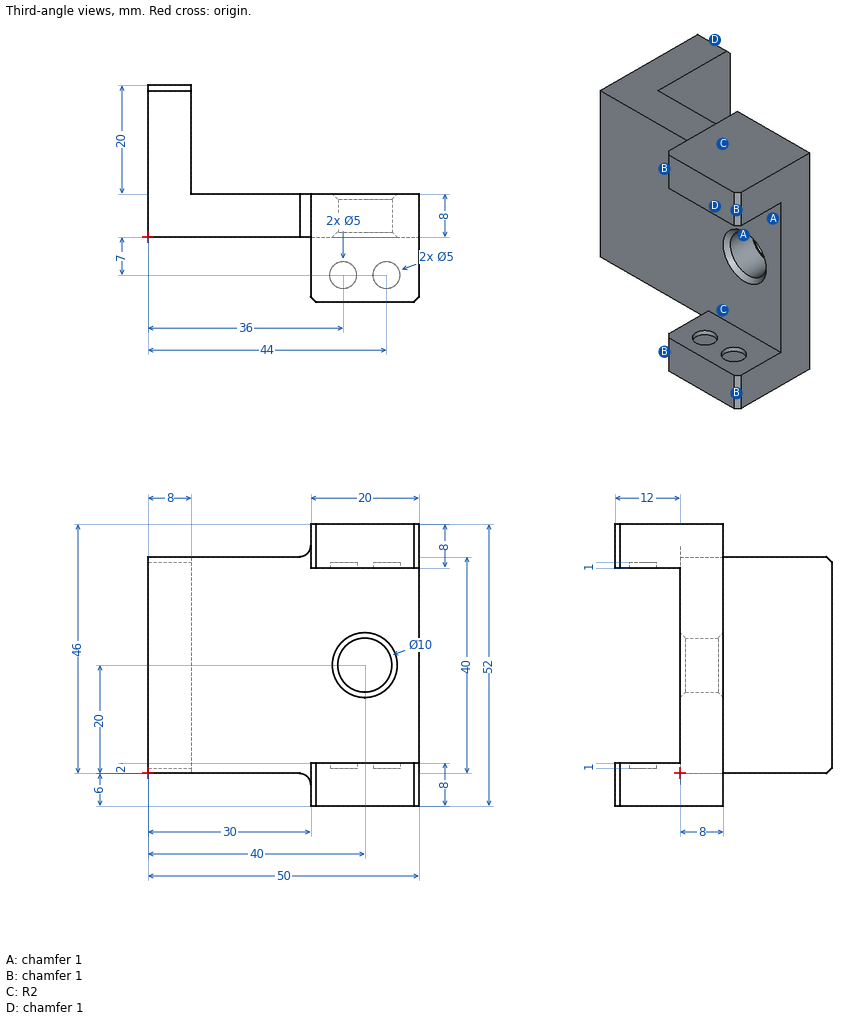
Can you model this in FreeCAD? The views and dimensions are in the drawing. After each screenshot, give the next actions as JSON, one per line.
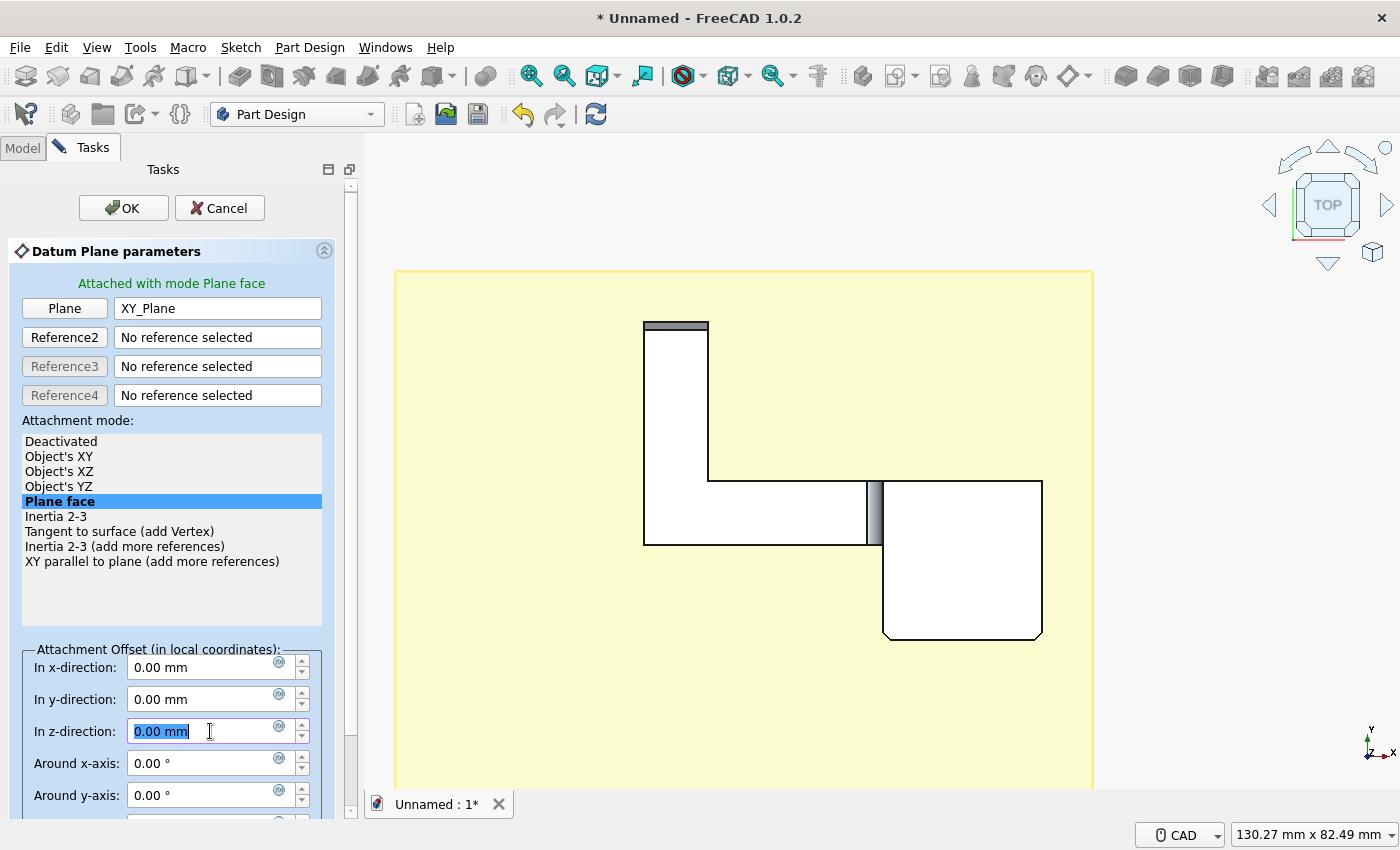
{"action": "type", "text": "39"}
{"action": "key", "text": "Tab"}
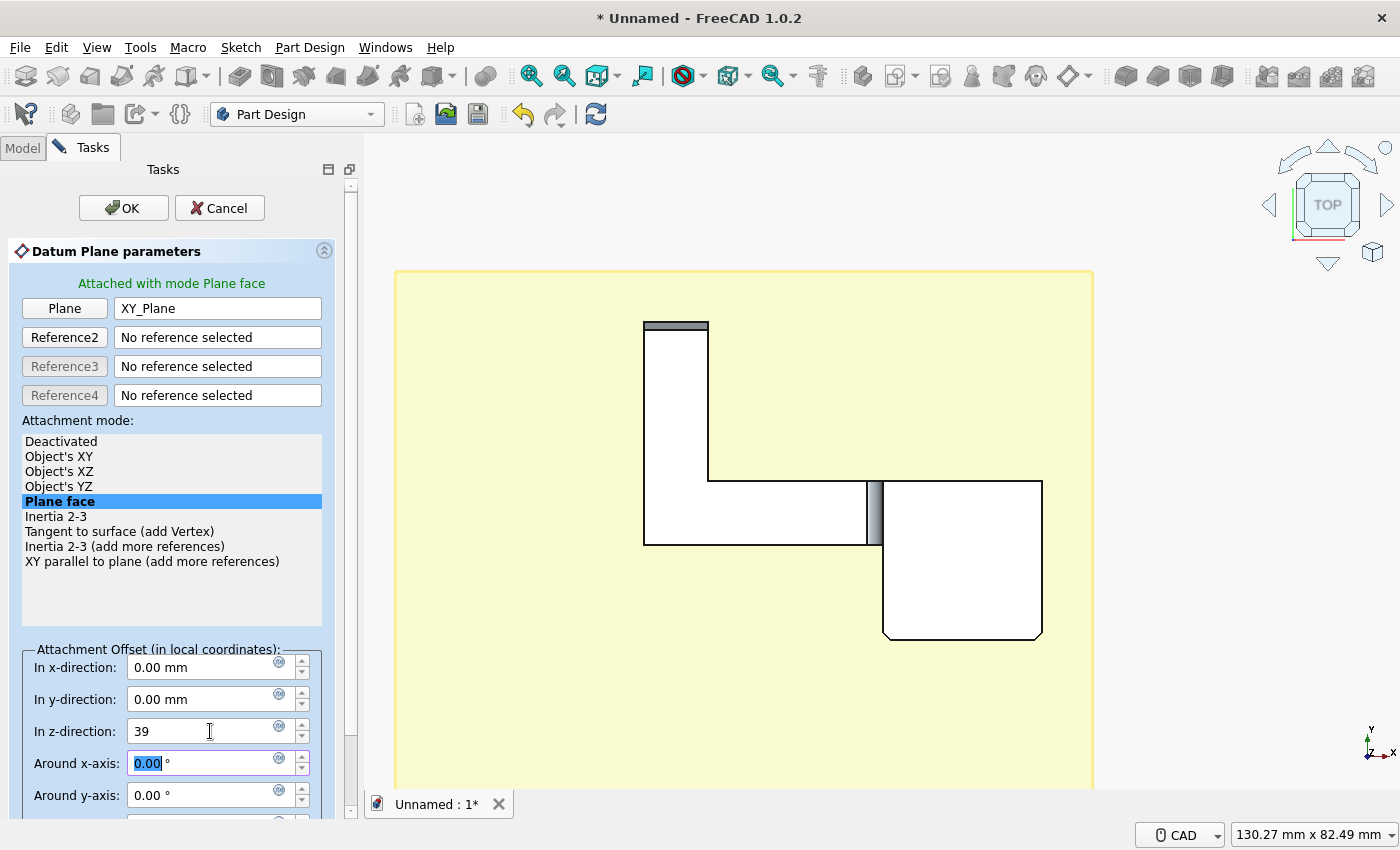
{"action": "left_click", "coordinate": [124, 208]}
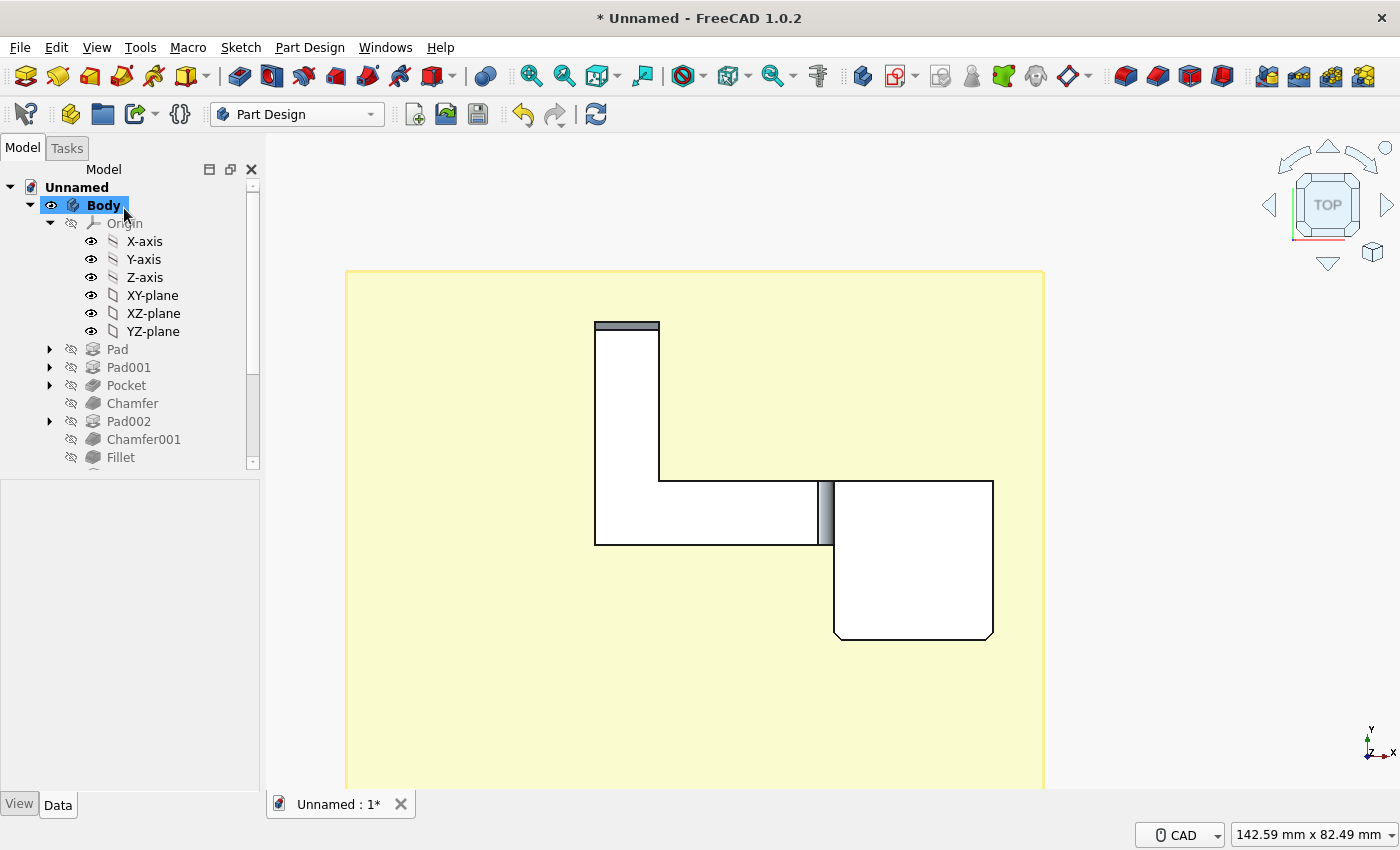
{"action": "scroll", "coordinate": [100, 327], "scroll_direction": "down", "scroll_amount": 3}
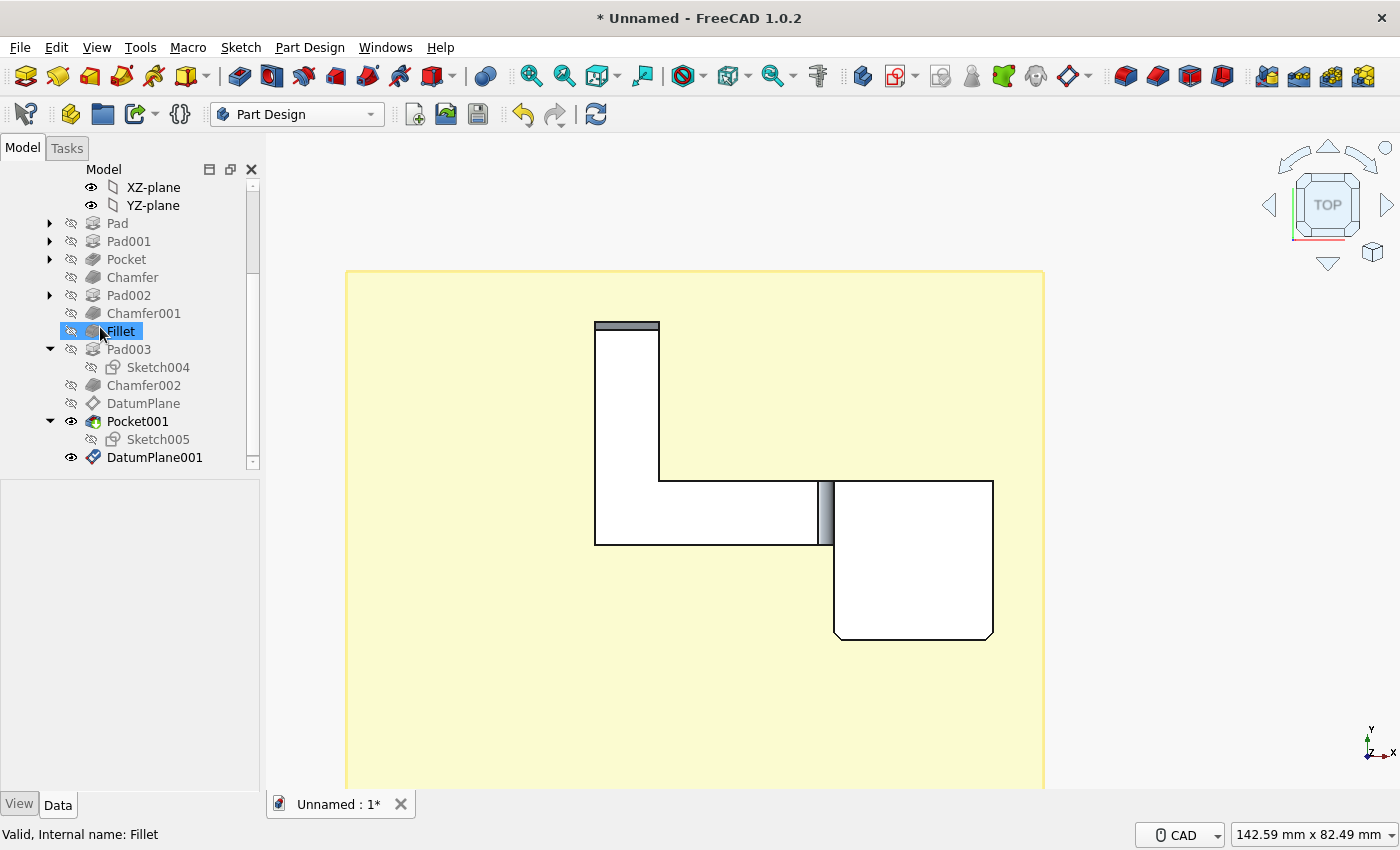
{"action": "left_click", "coordinate": [116, 457]}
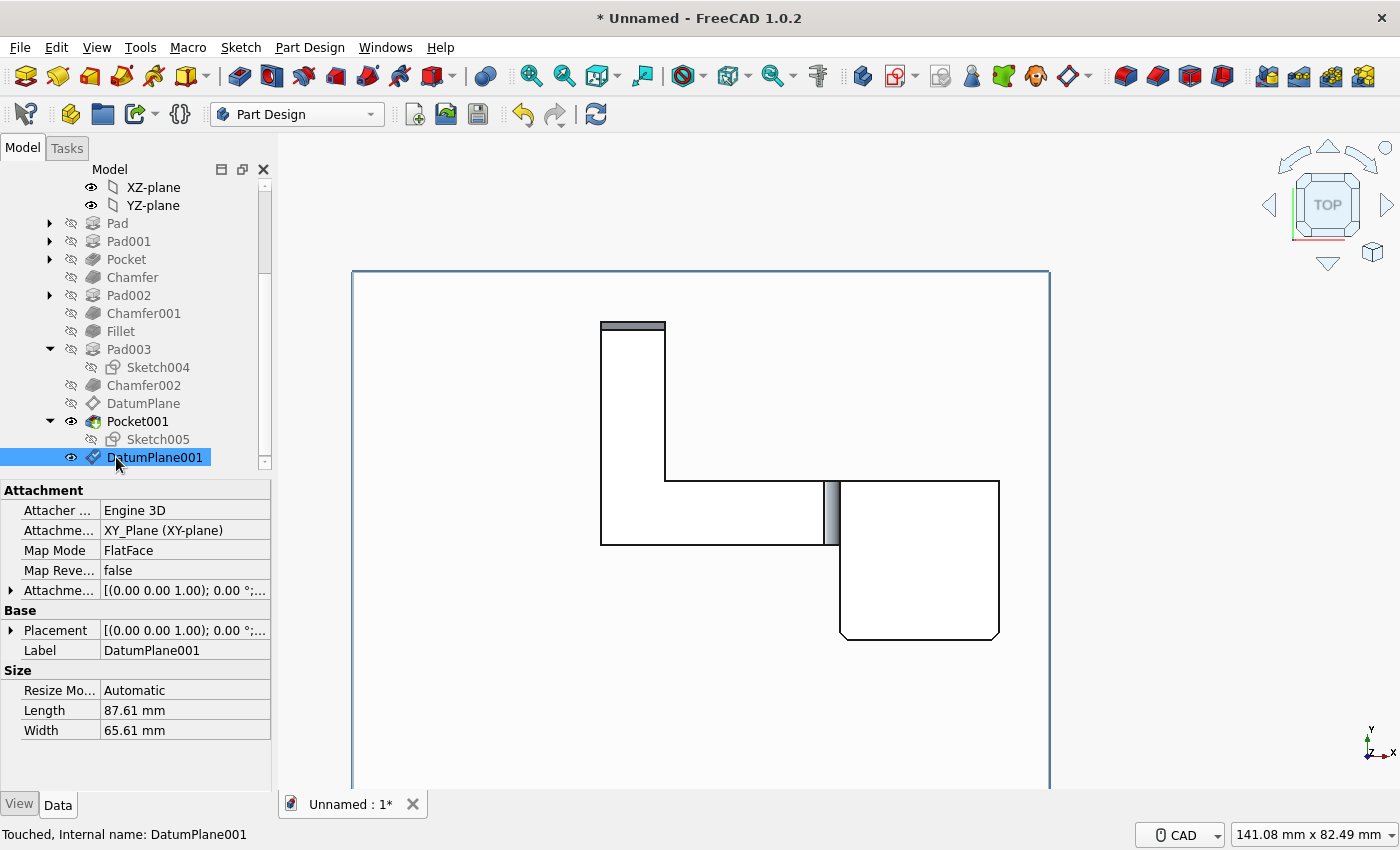
{"action": "left_click", "coordinate": [896, 76]}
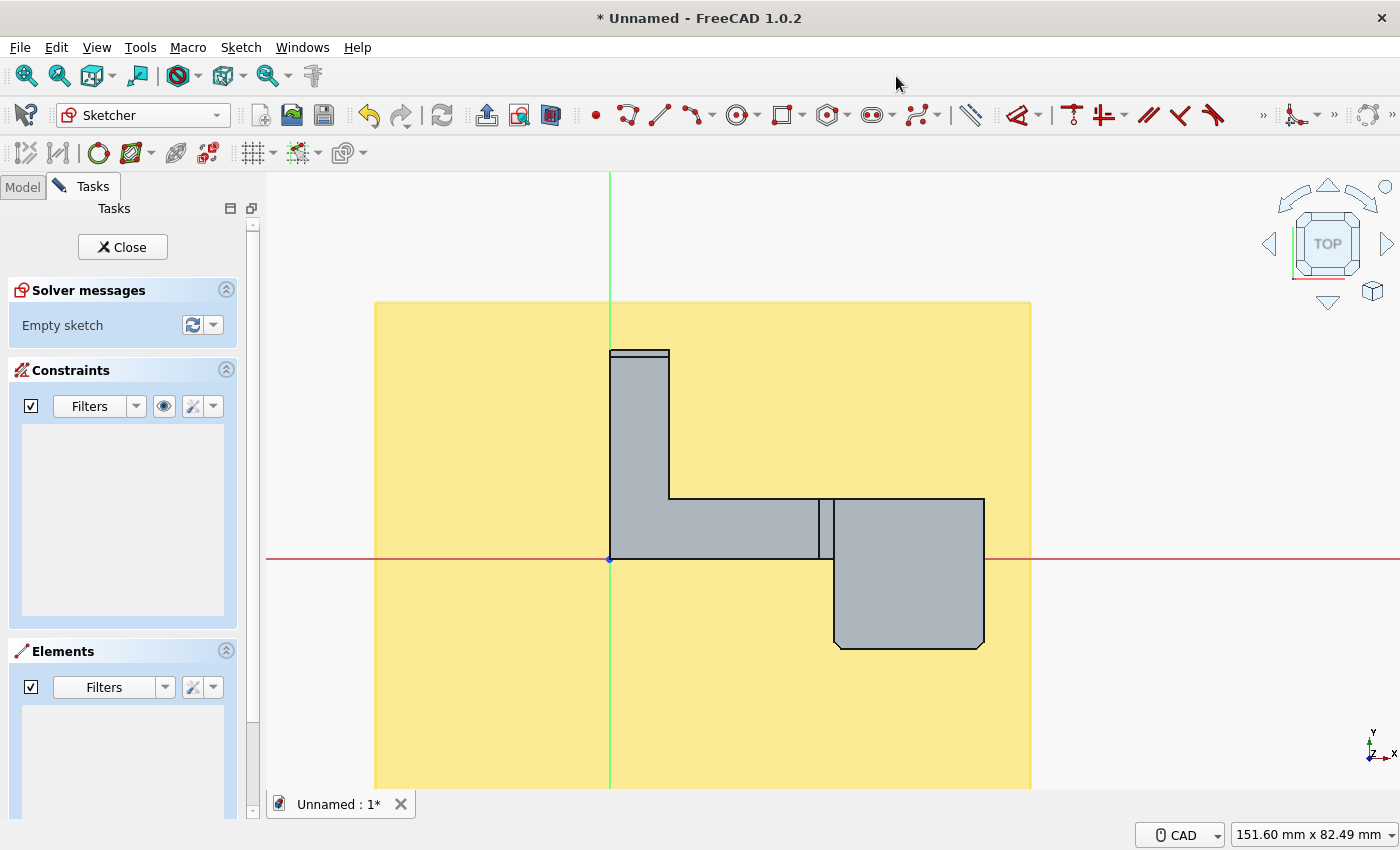
{"action": "left_click", "coordinate": [552, 116]}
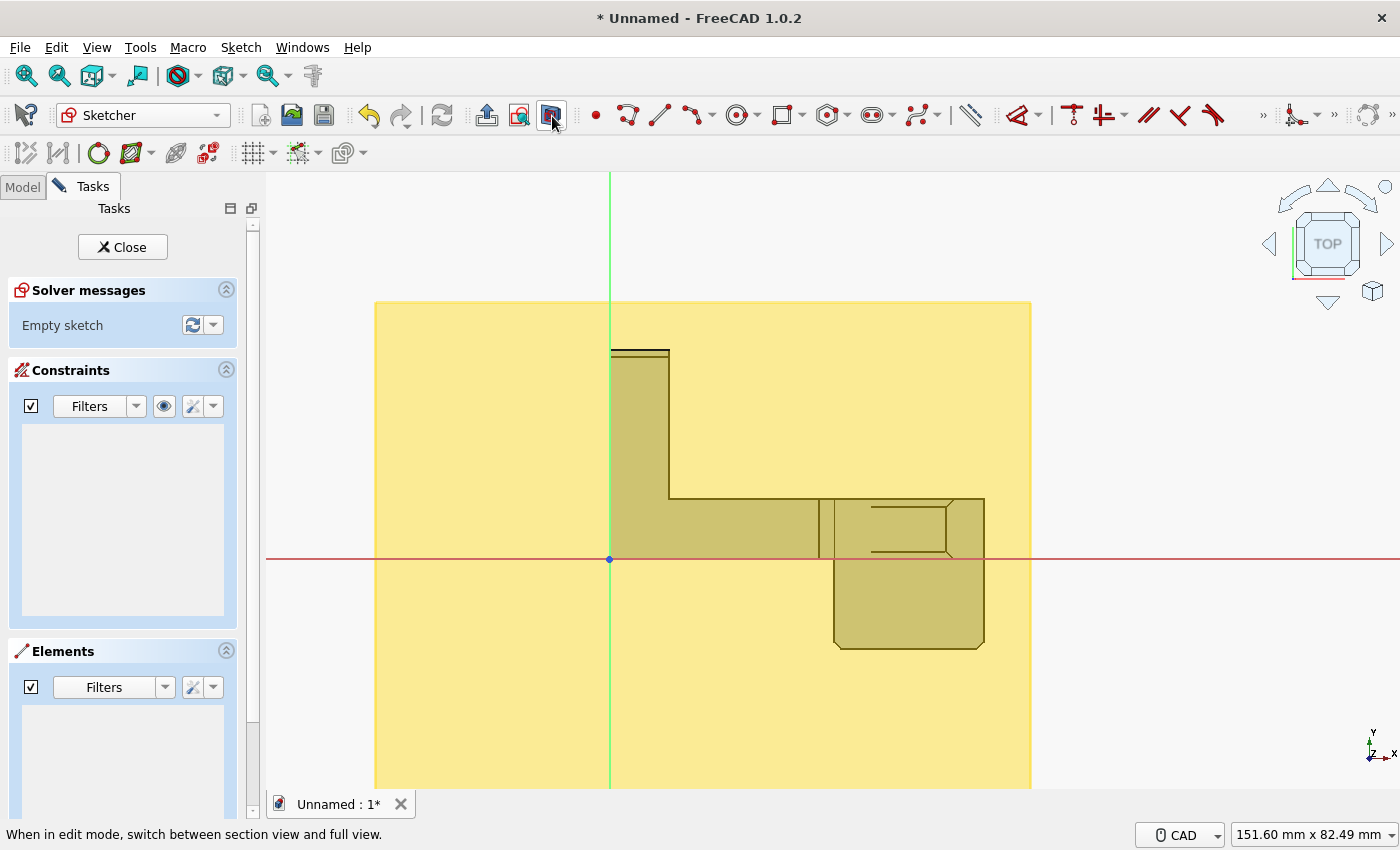
{"action": "scroll", "coordinate": [931, 632], "scroll_direction": "up", "scroll_amount": 10}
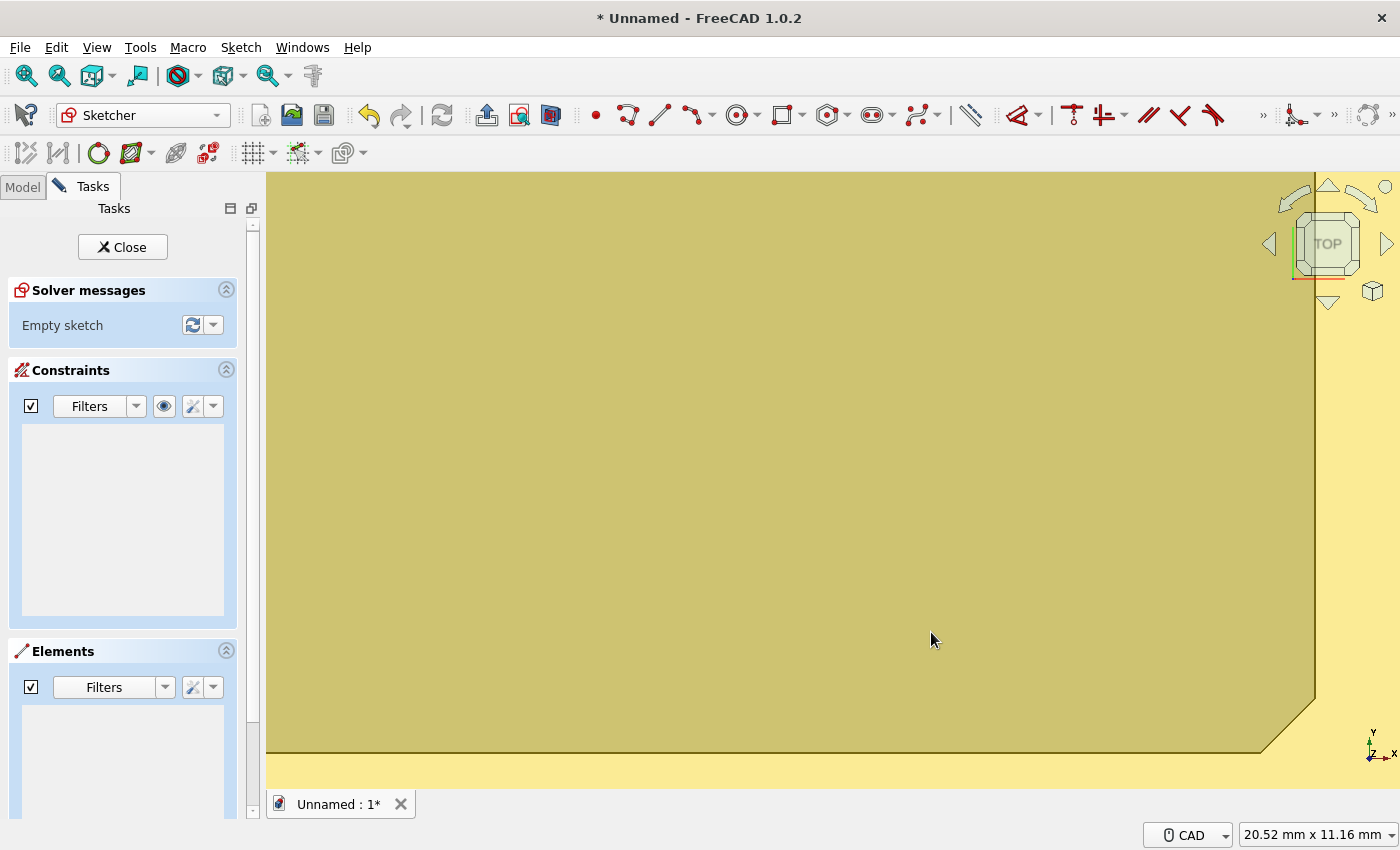
{"action": "left_click", "coordinate": [738, 116]}